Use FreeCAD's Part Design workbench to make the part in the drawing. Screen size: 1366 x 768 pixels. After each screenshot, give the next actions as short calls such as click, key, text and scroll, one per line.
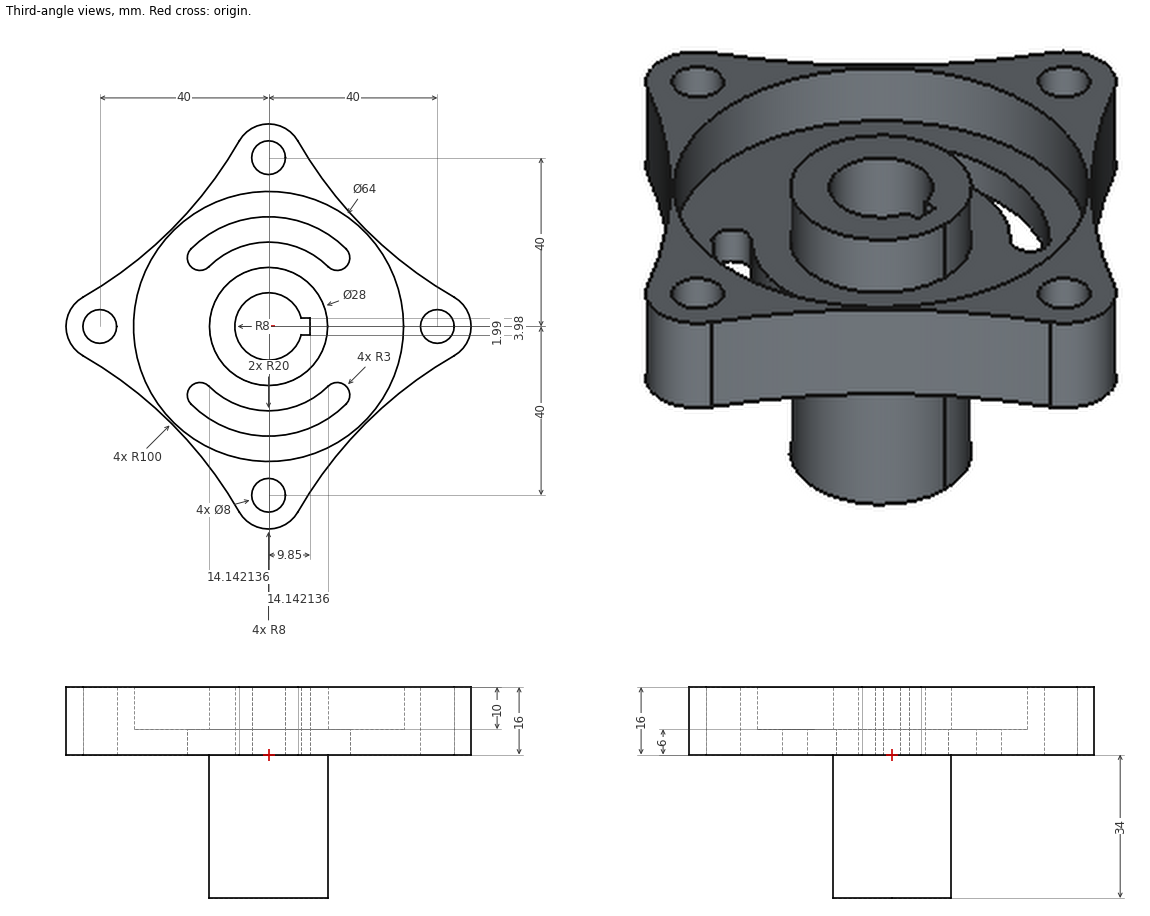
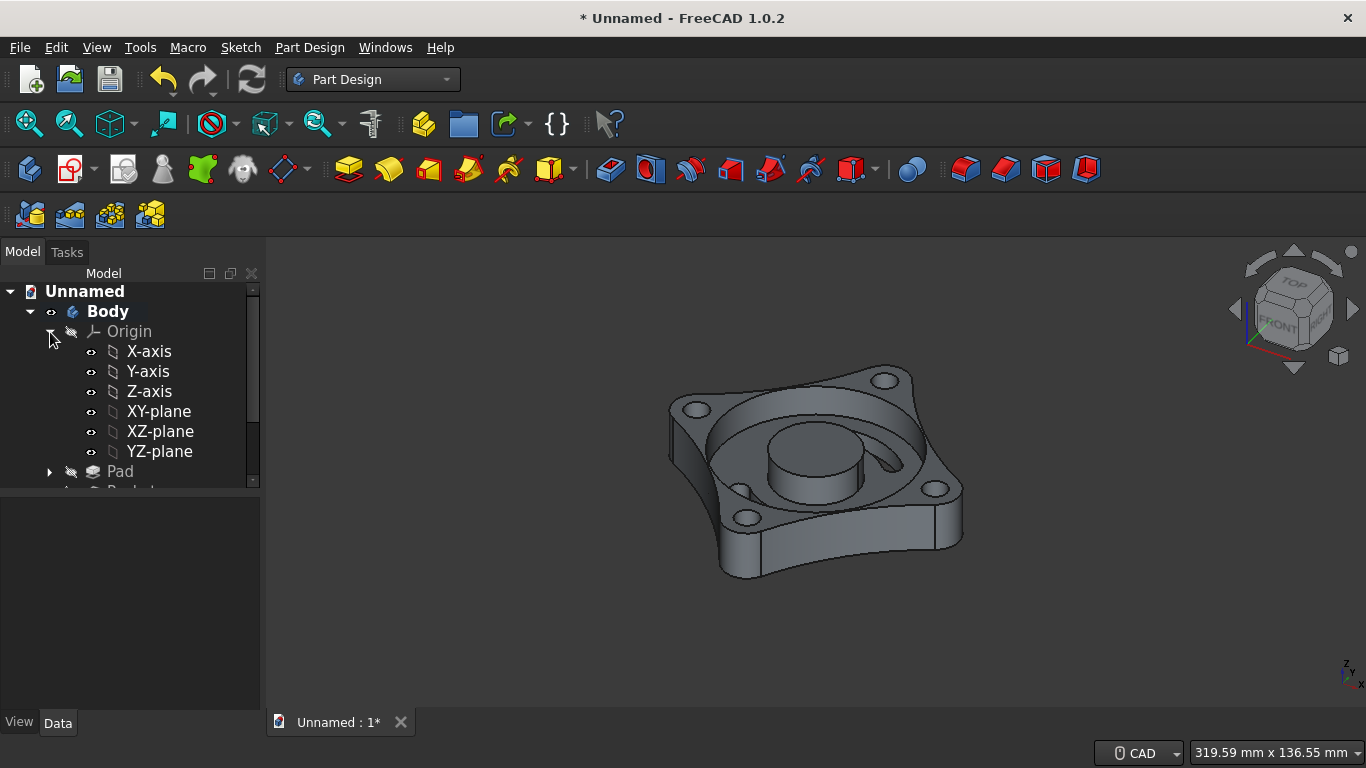
click(136, 412)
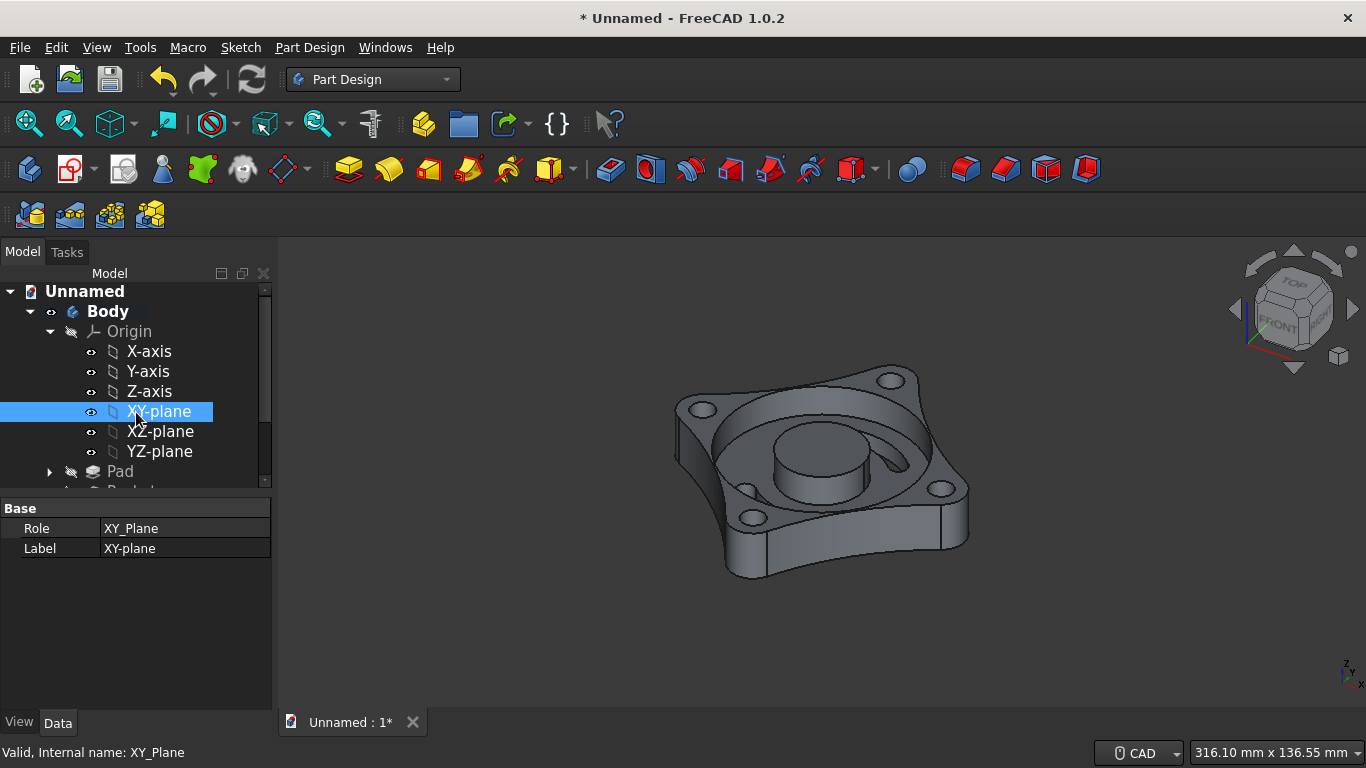
click(284, 170)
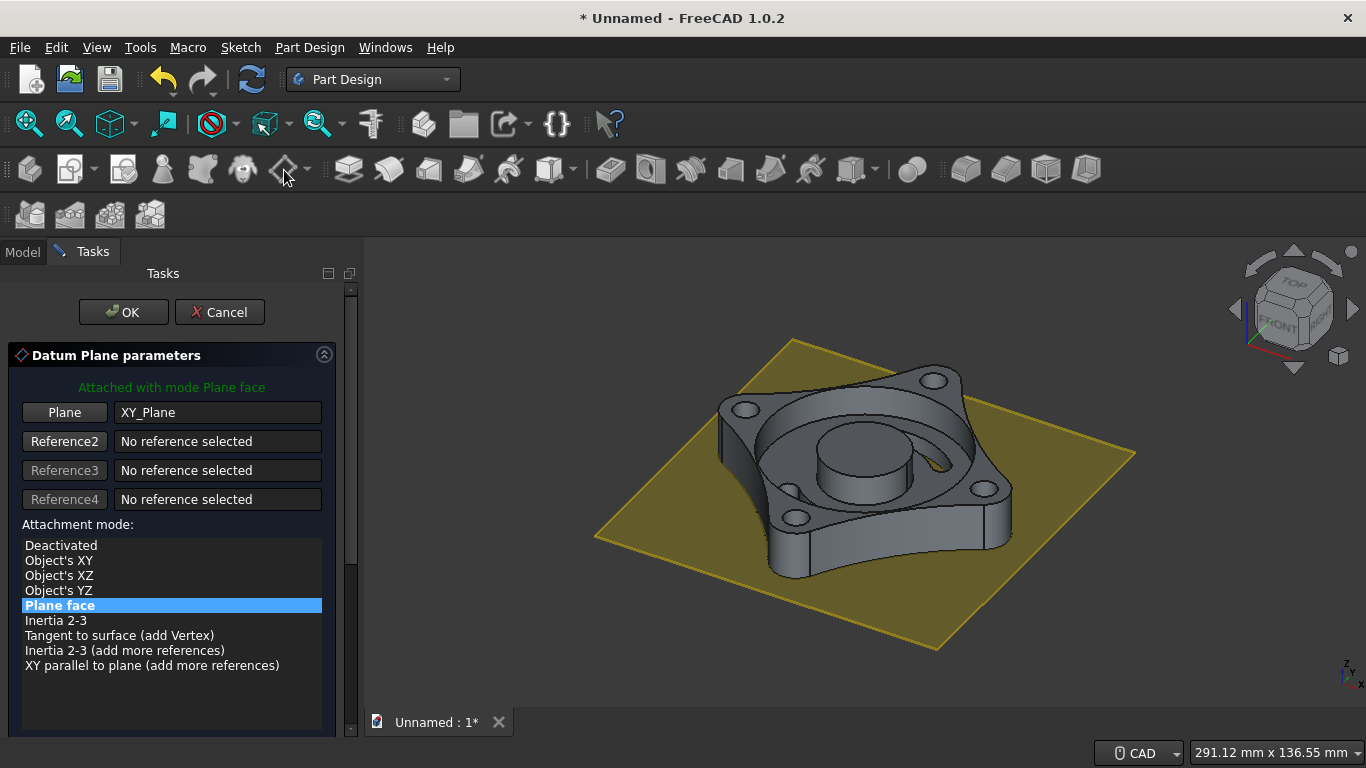
scroll(351, 510, down, 3)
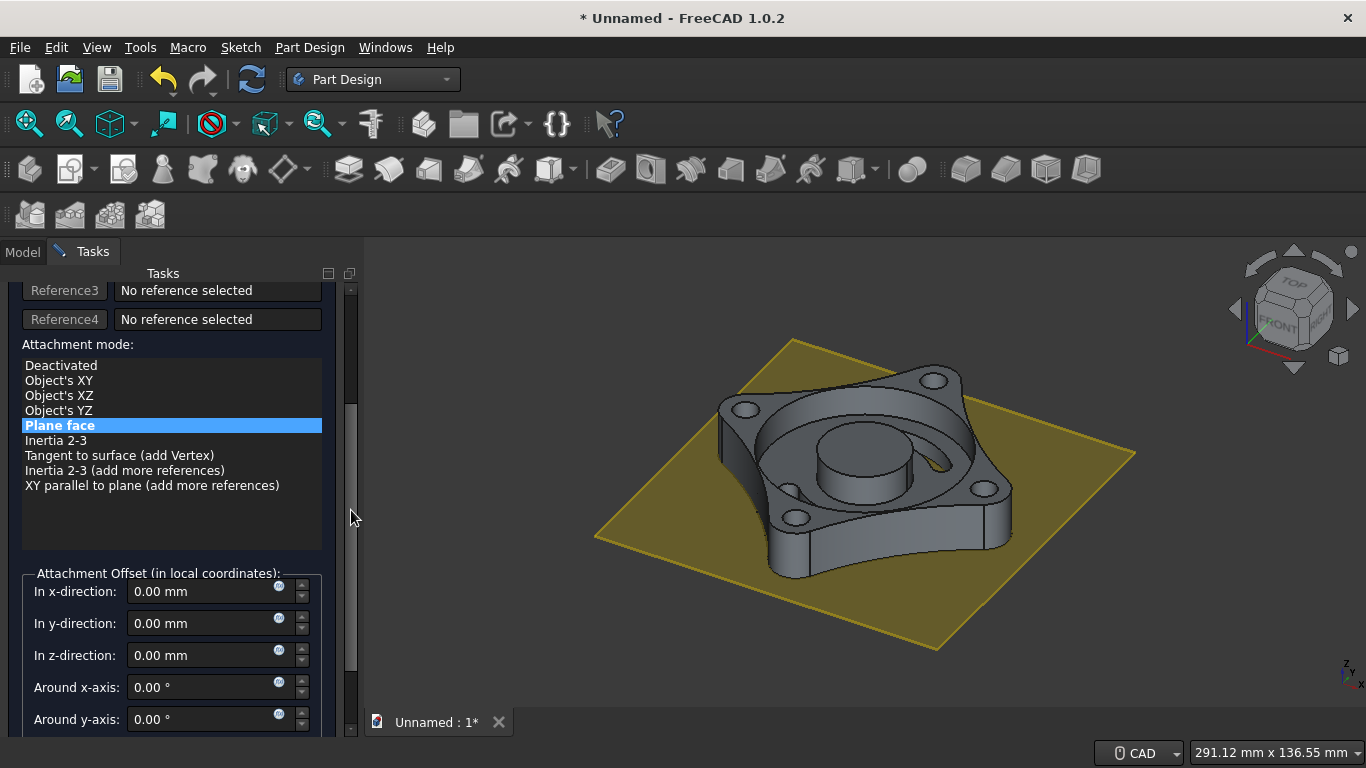
triple_click(210, 655)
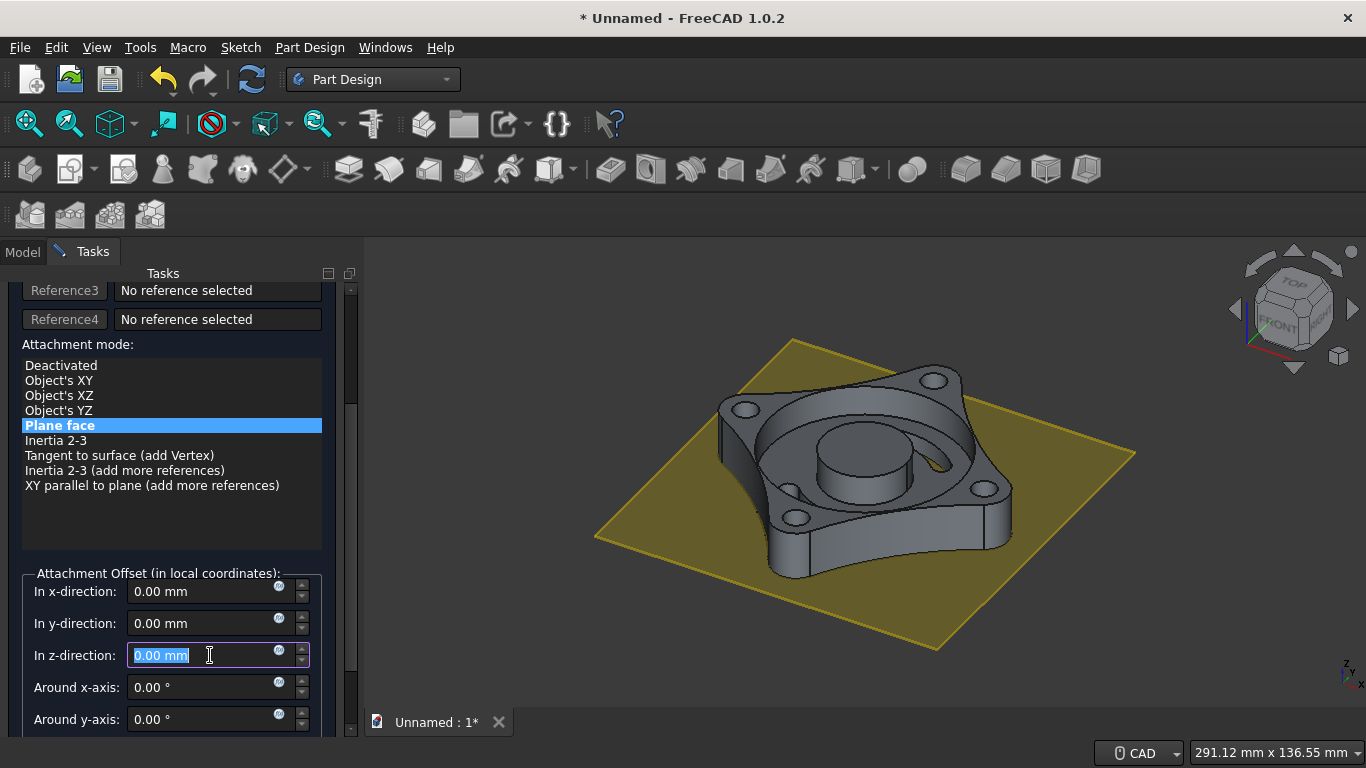
text(-34)
key(Tab)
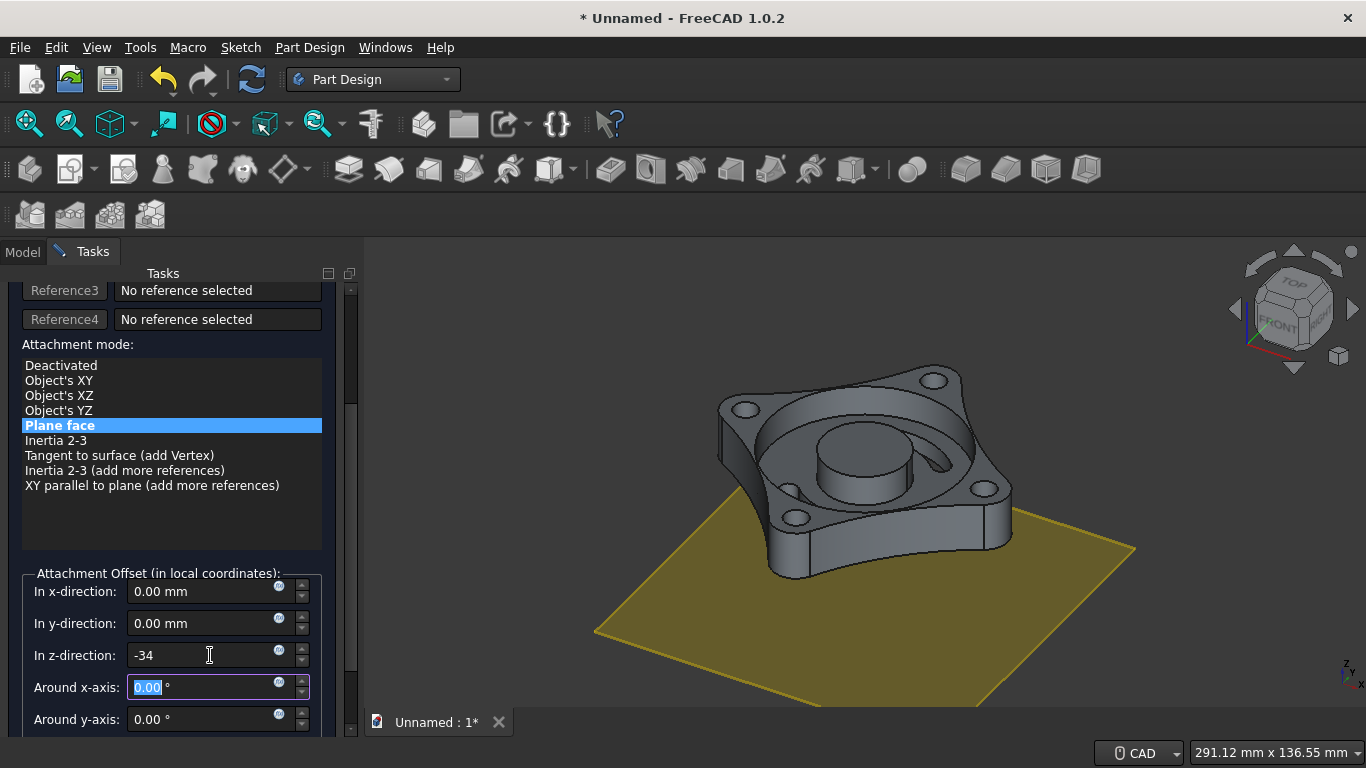
scroll(351, 510, up, 4)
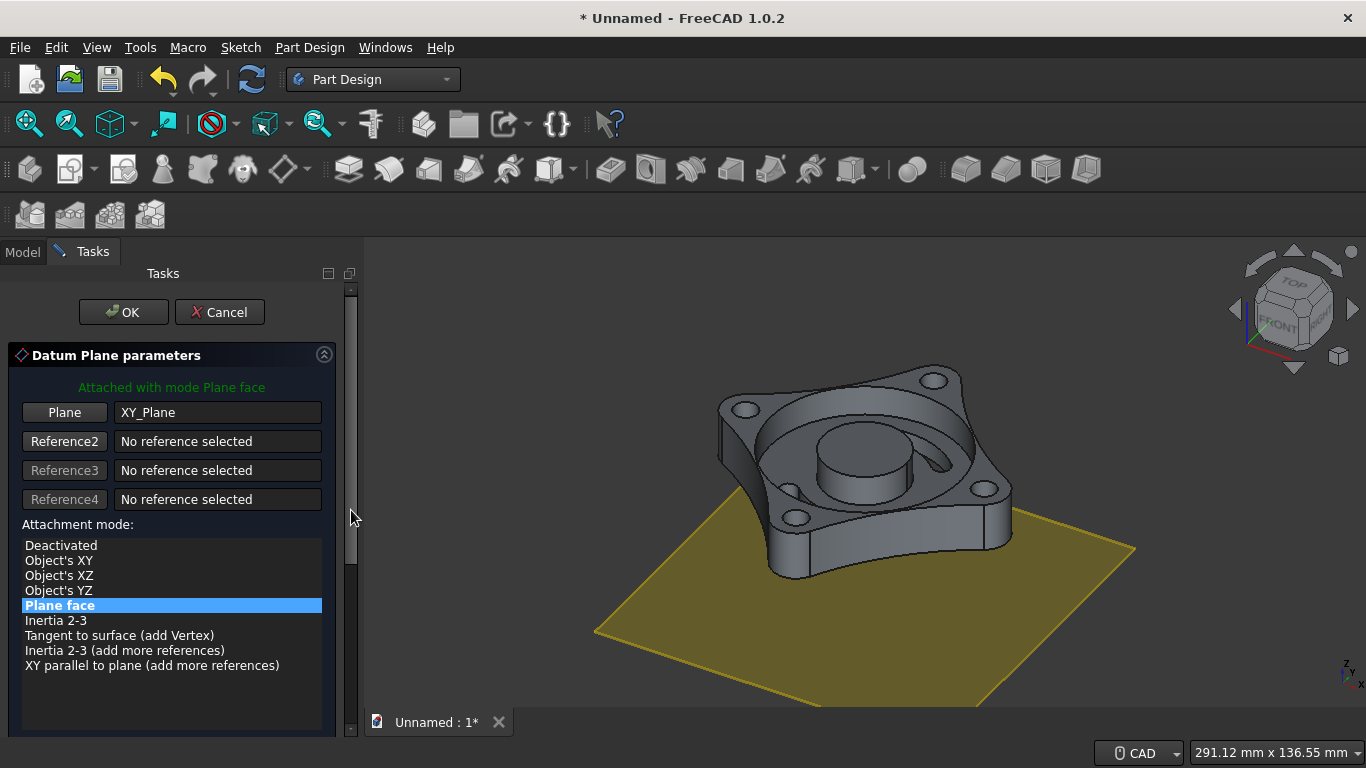
click(124, 312)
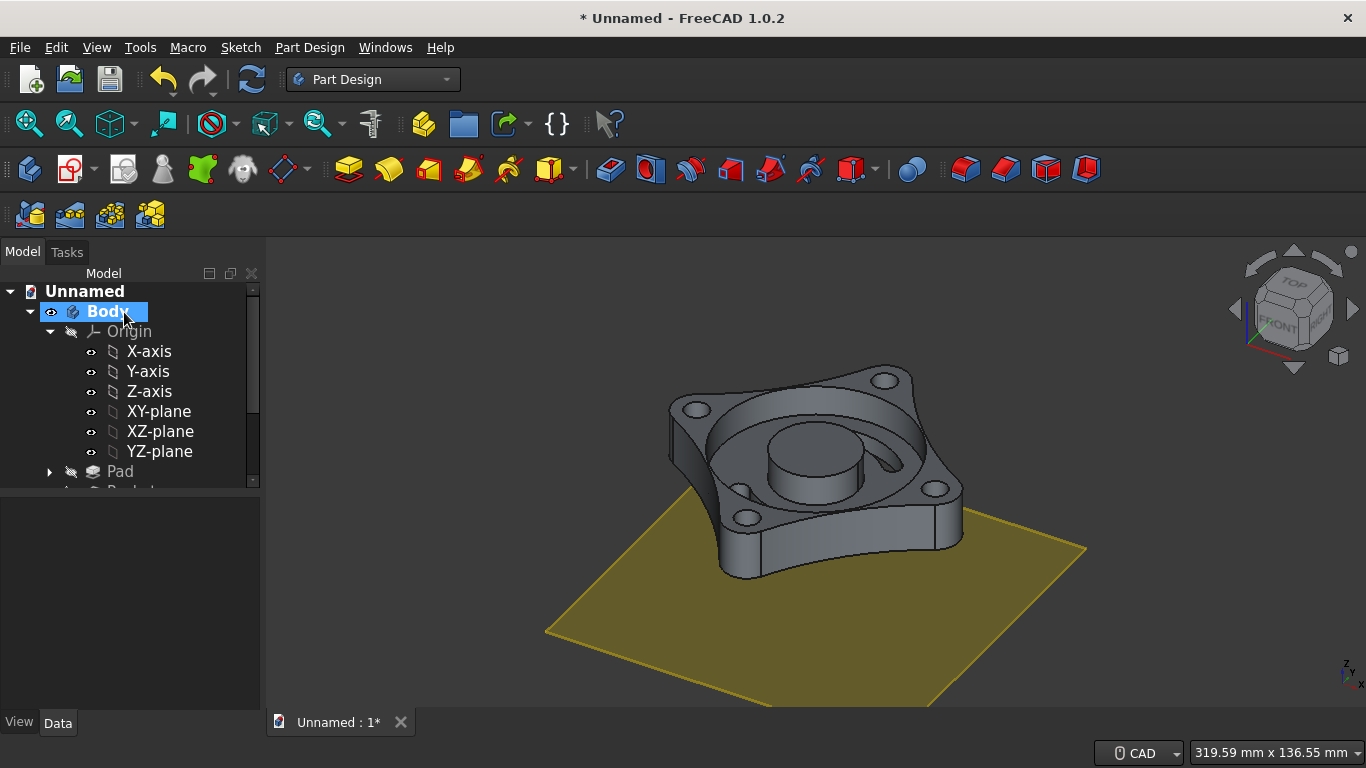
scroll(100, 387, down, 3)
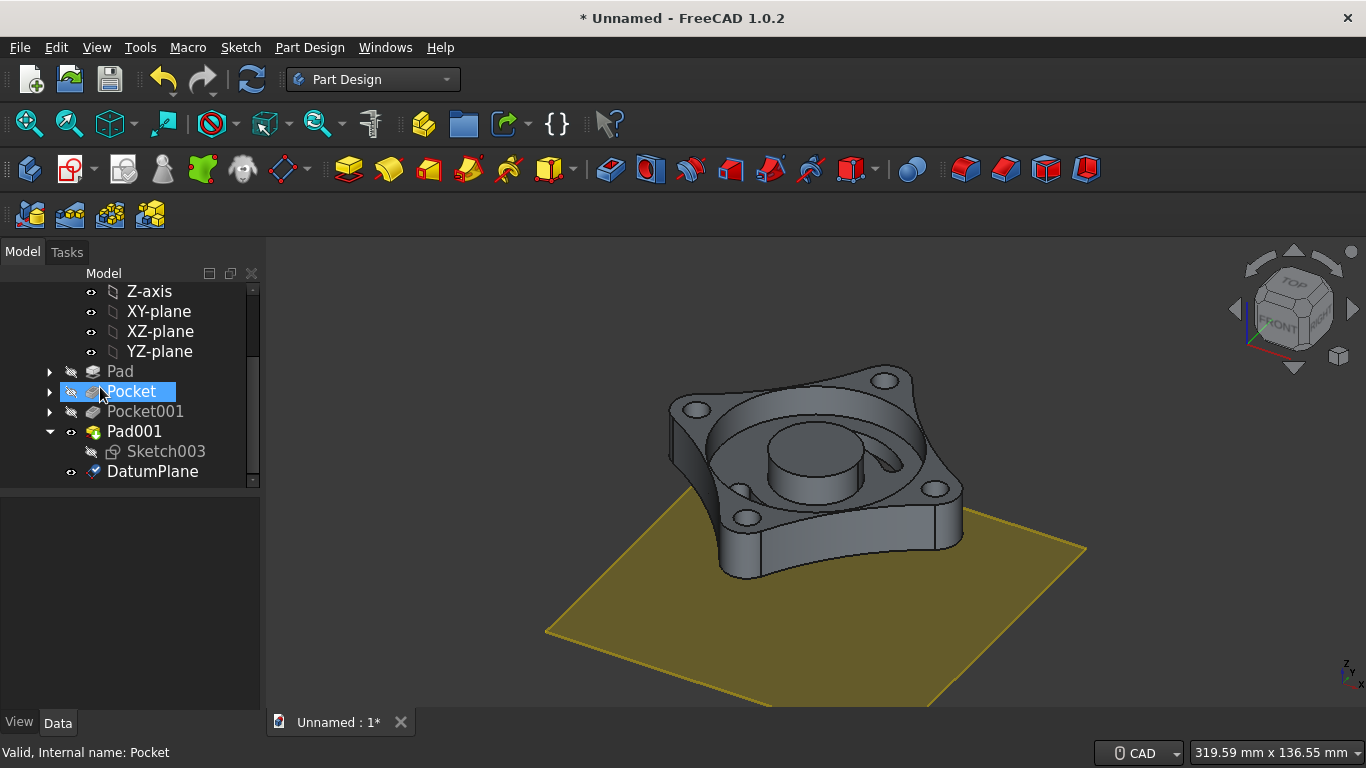
click(116, 472)